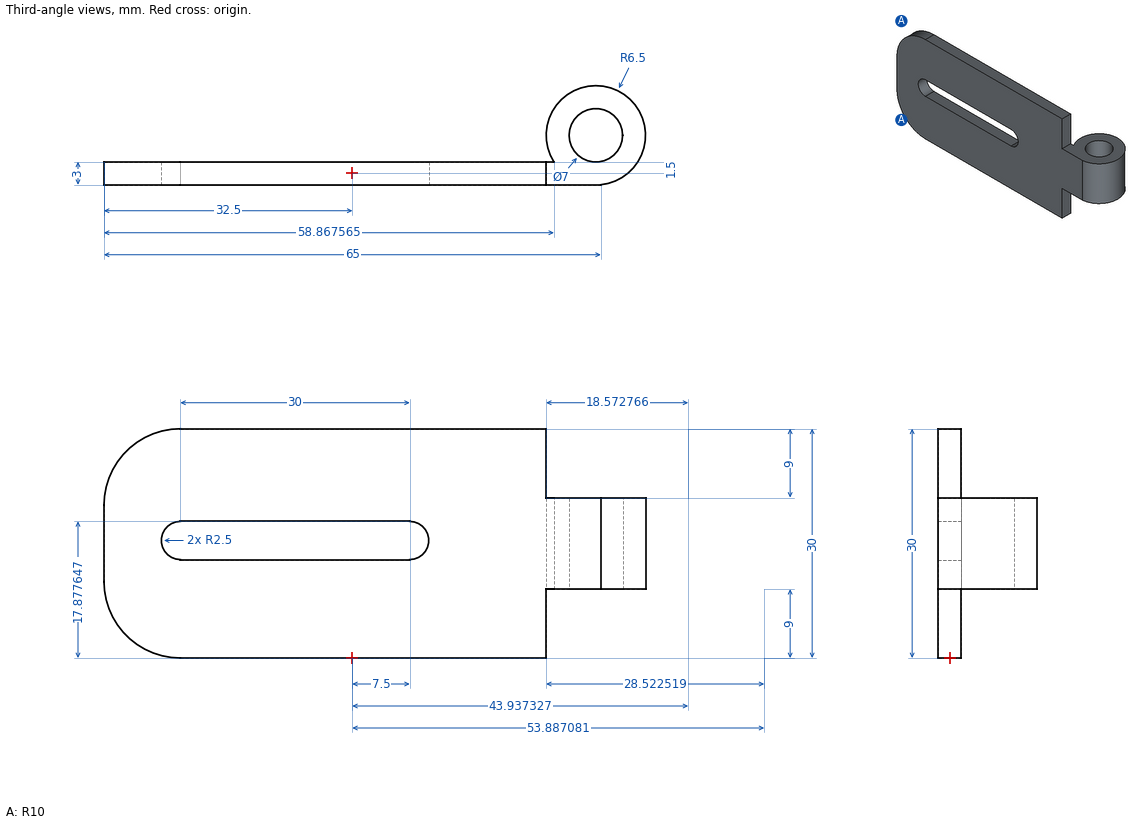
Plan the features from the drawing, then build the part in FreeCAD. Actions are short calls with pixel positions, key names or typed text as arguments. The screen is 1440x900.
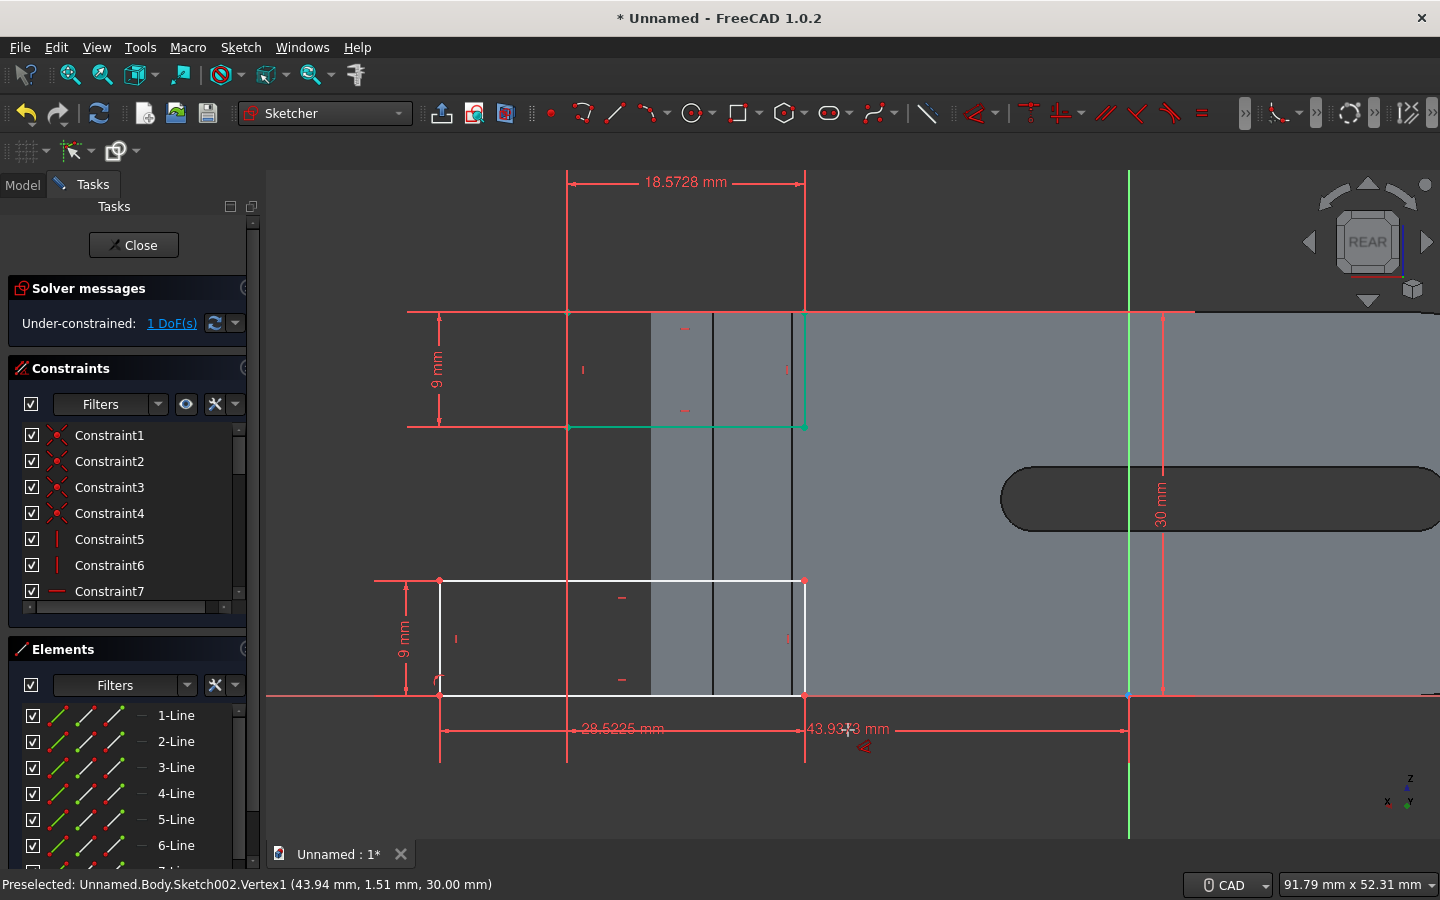
click(440, 581)
click(943, 730)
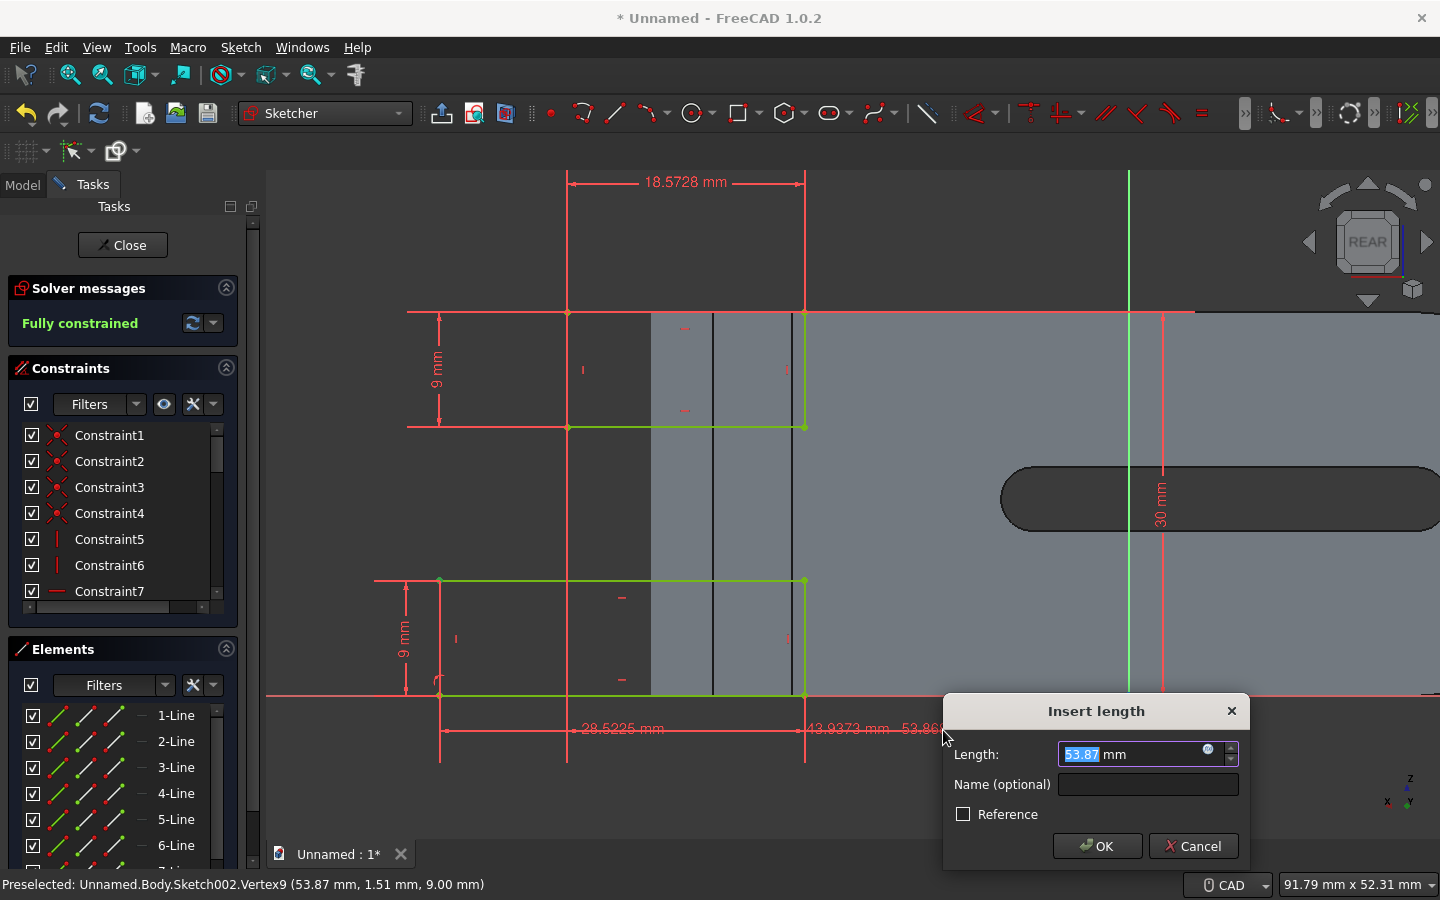
text(53.887081)
key(Return)
key(Escape)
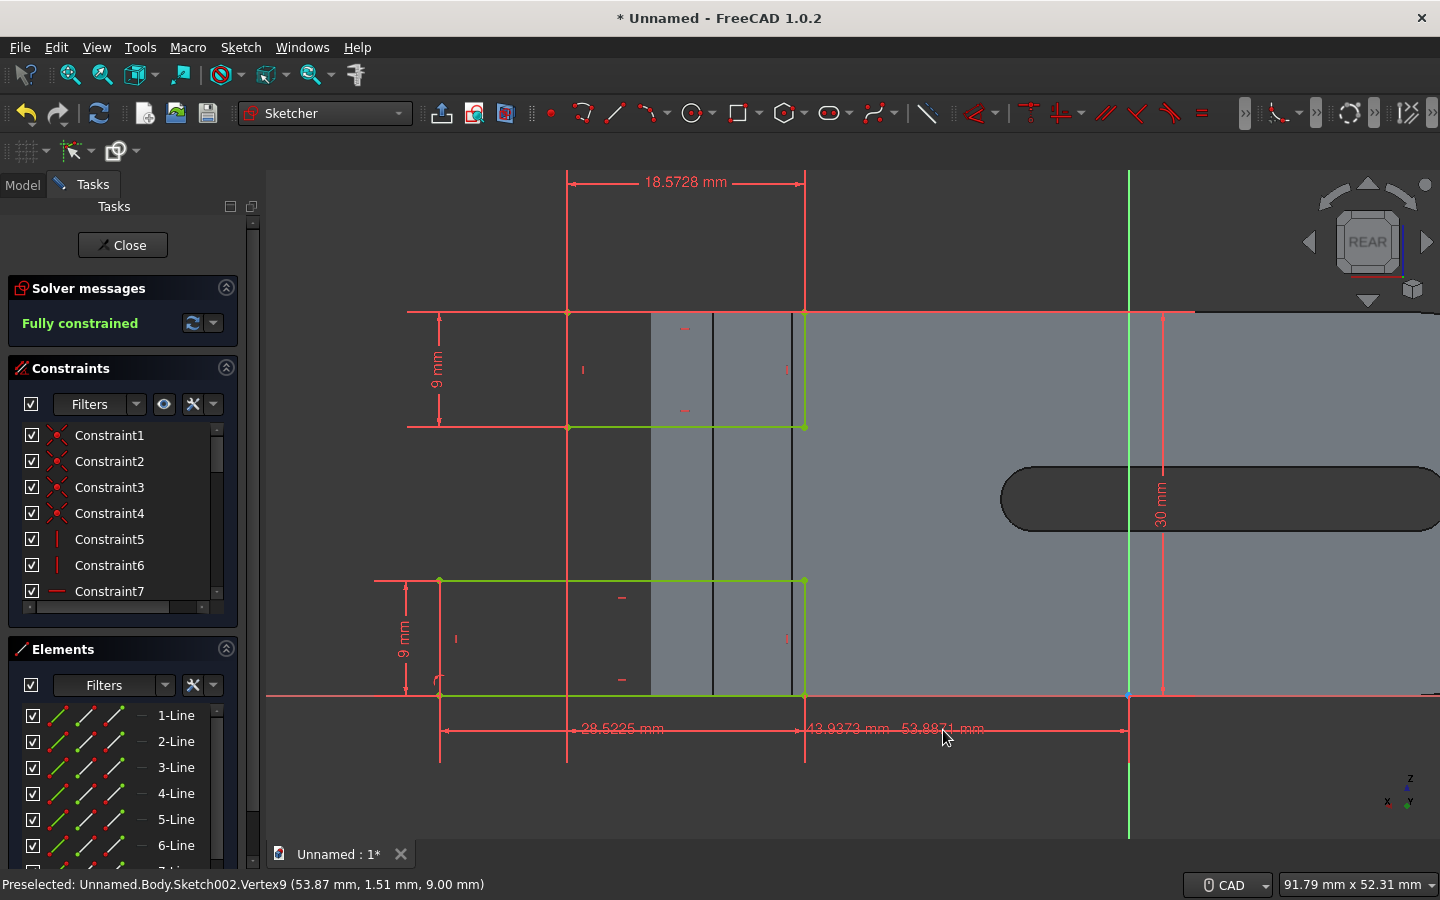
click(123, 245)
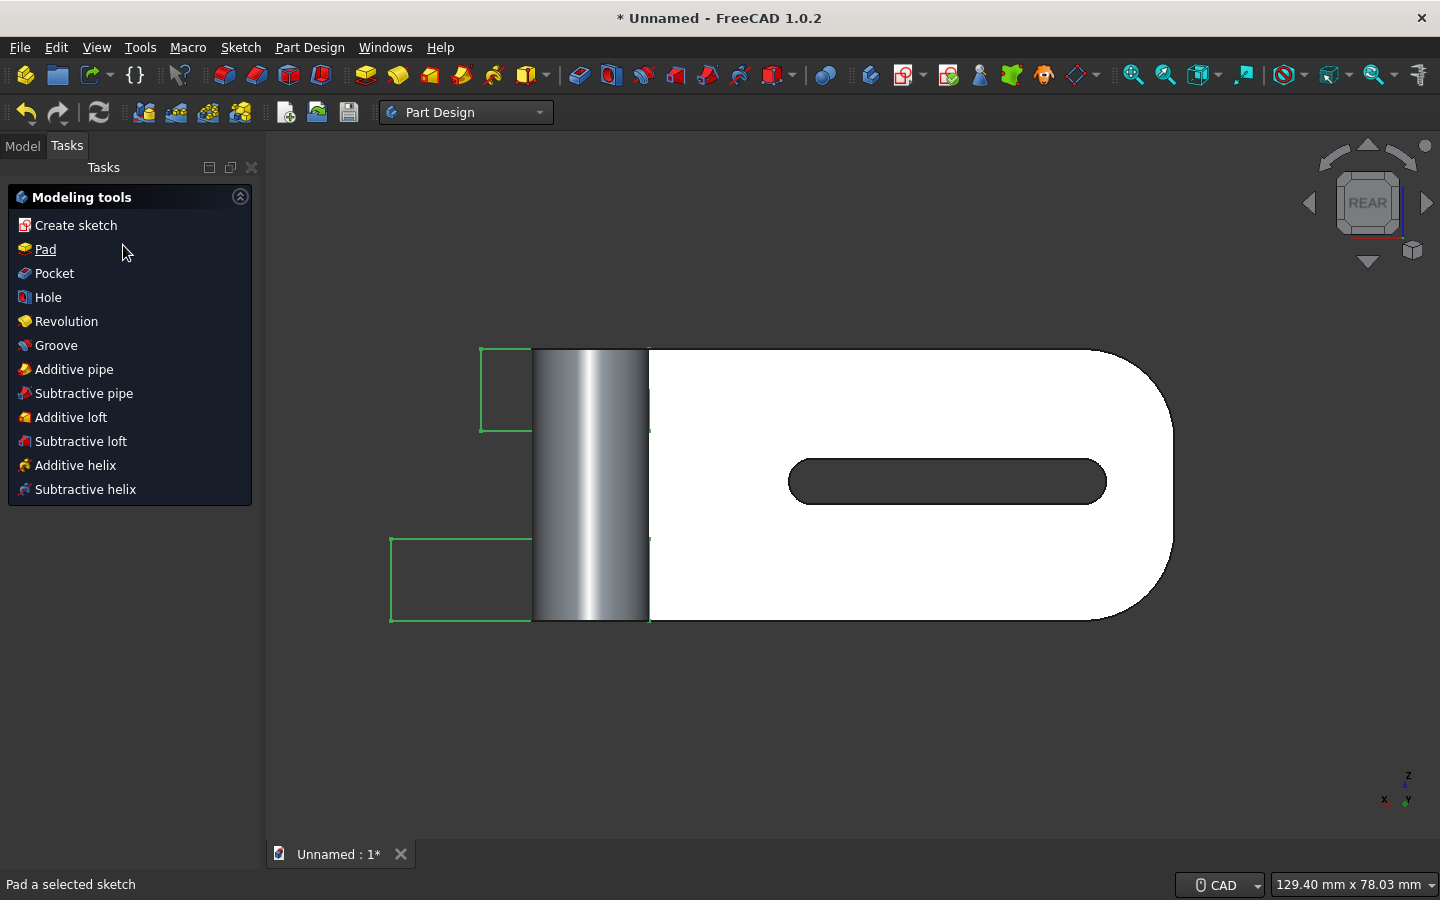
click(580, 76)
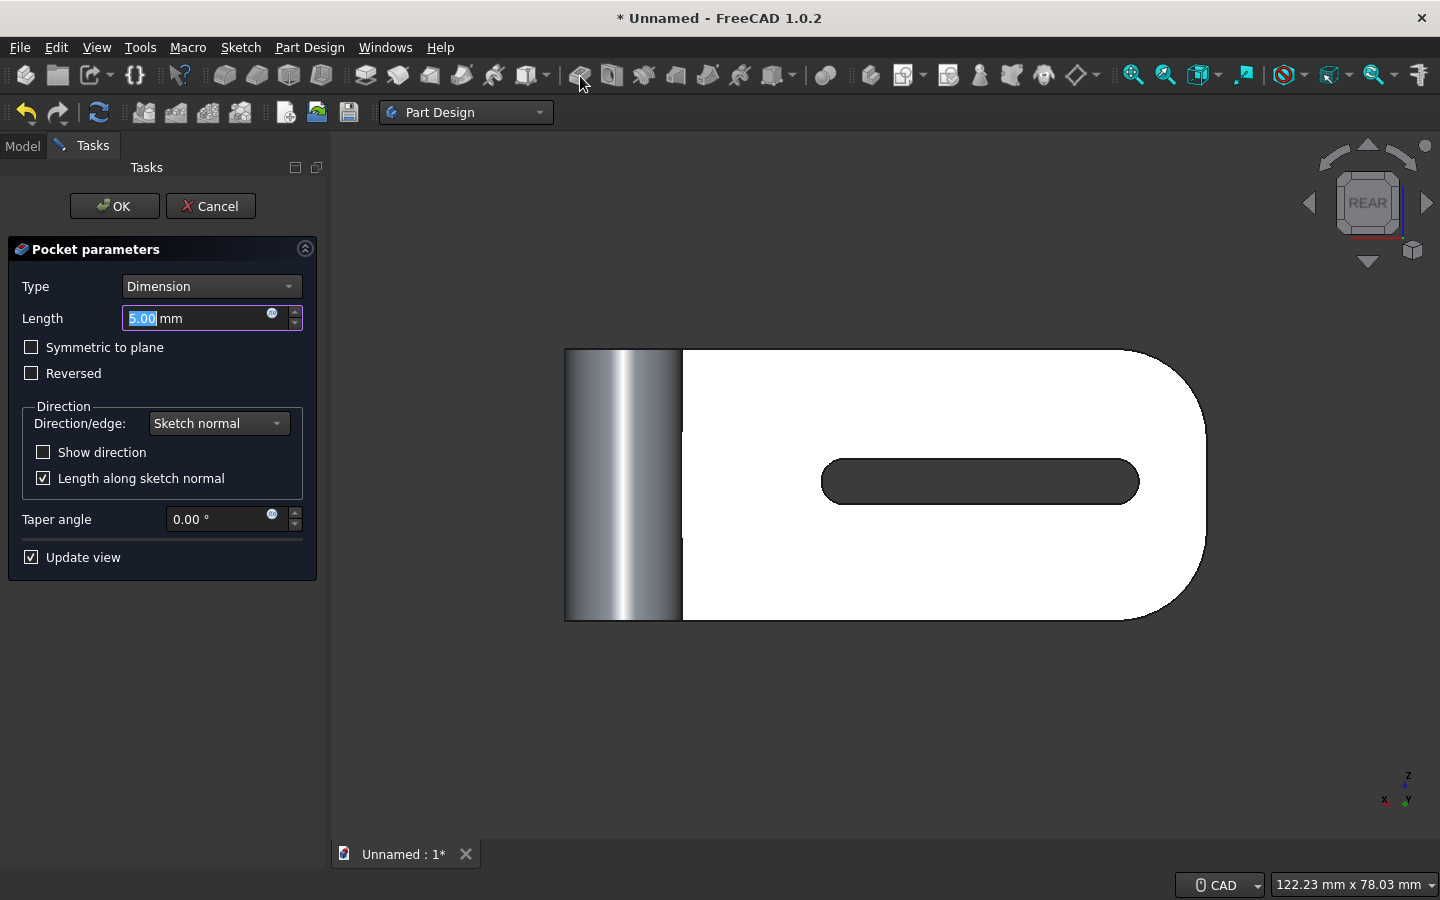
text(30)
key(Tab)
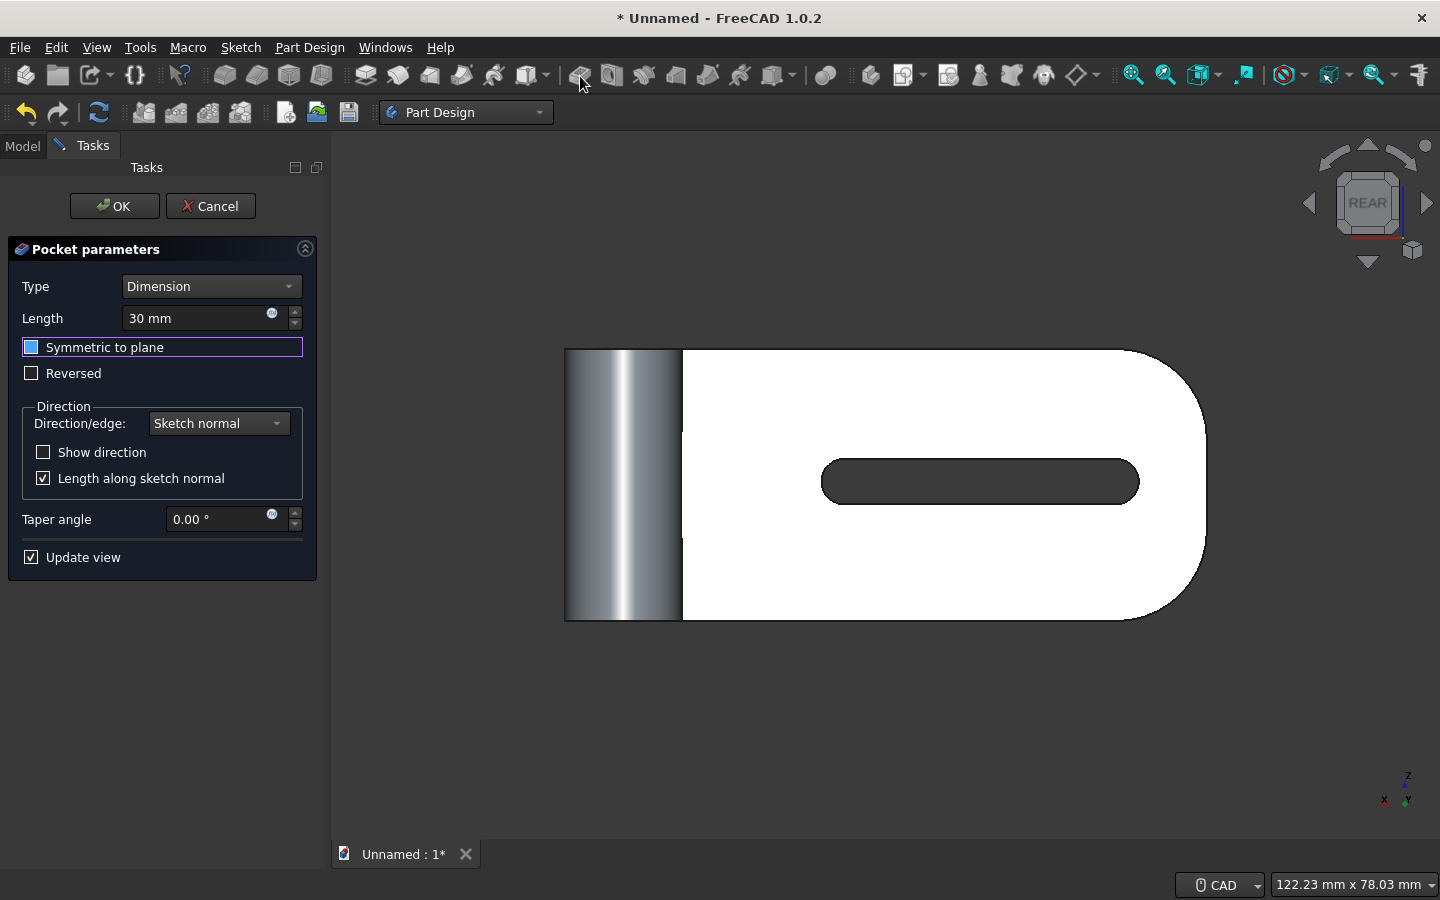
click(30, 347)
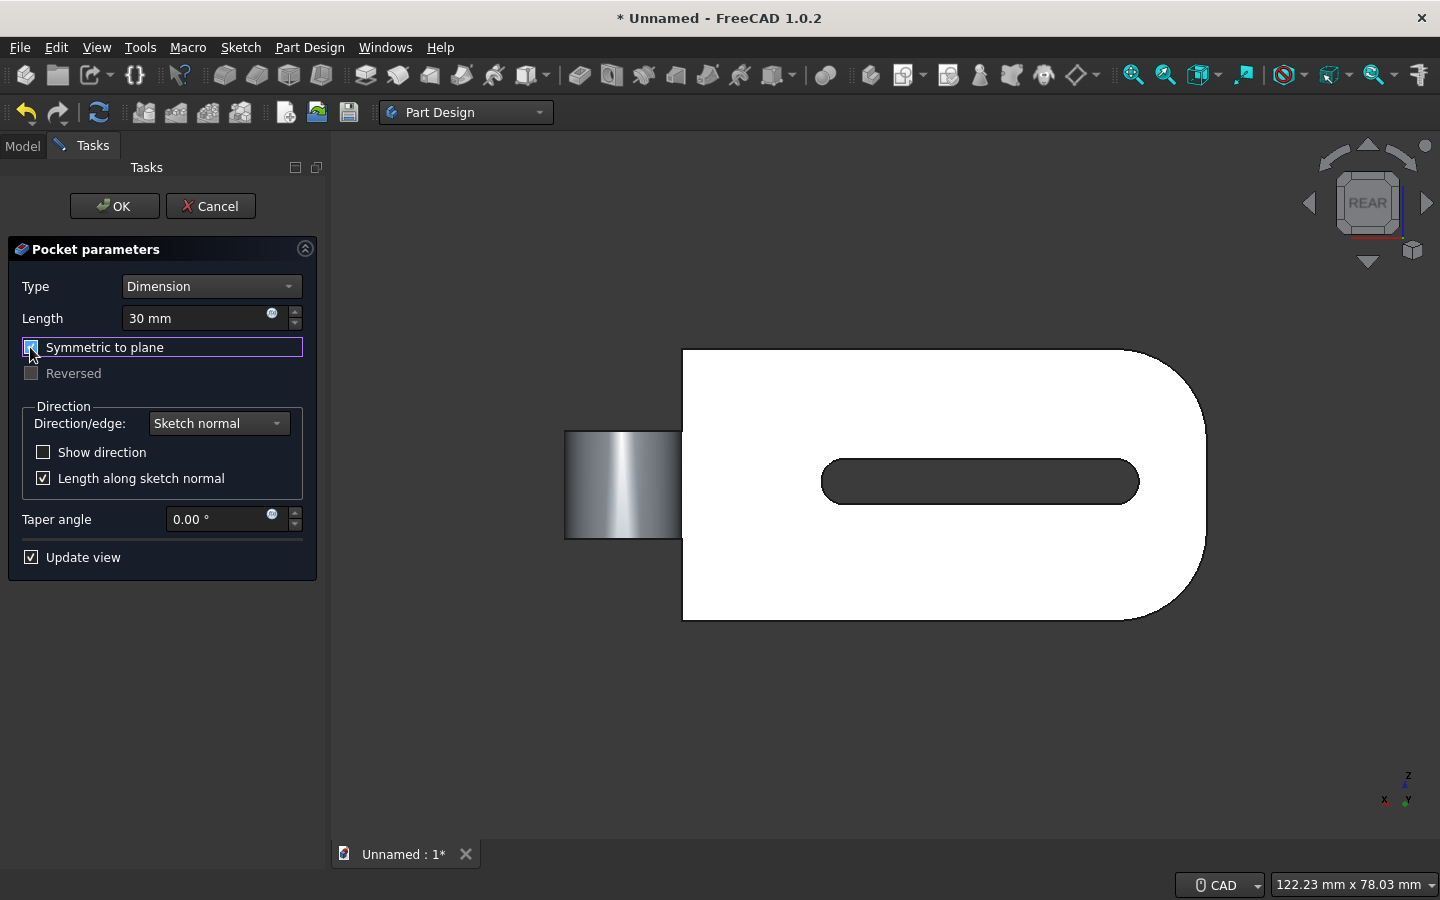
click(115, 206)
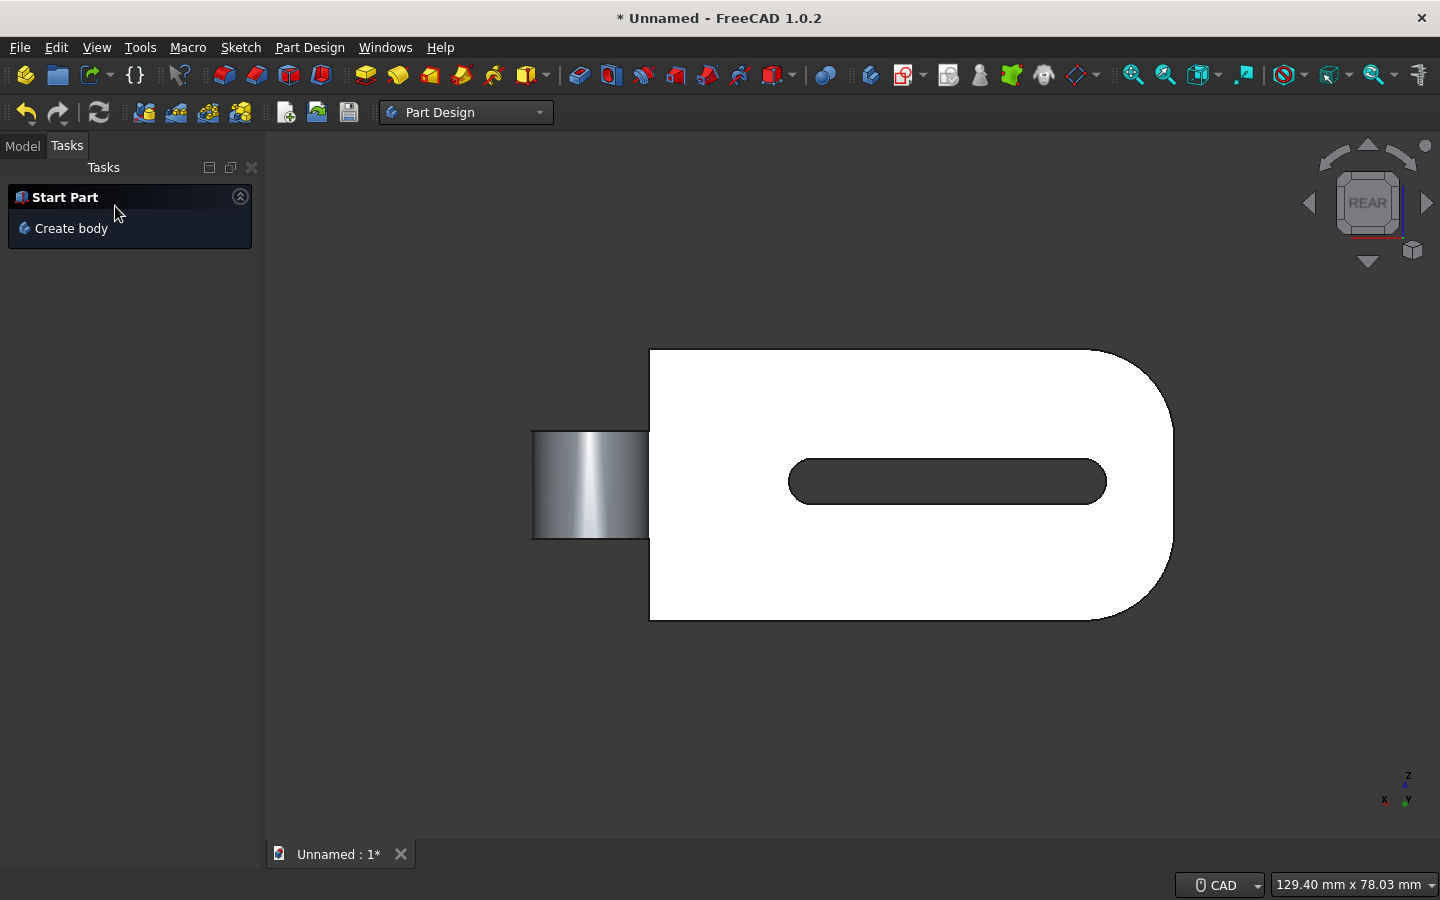
key(0)